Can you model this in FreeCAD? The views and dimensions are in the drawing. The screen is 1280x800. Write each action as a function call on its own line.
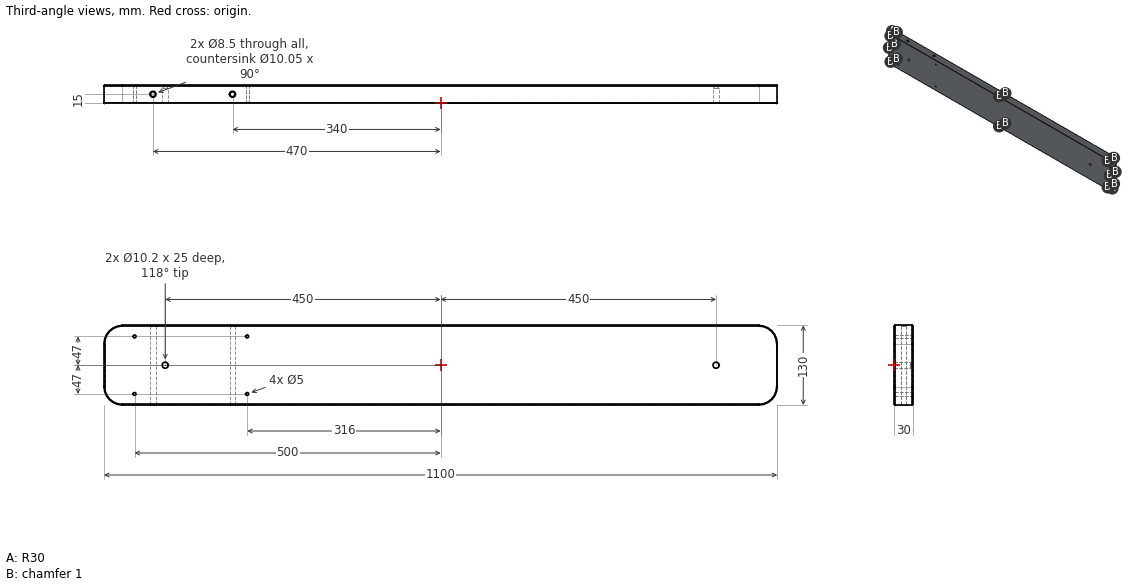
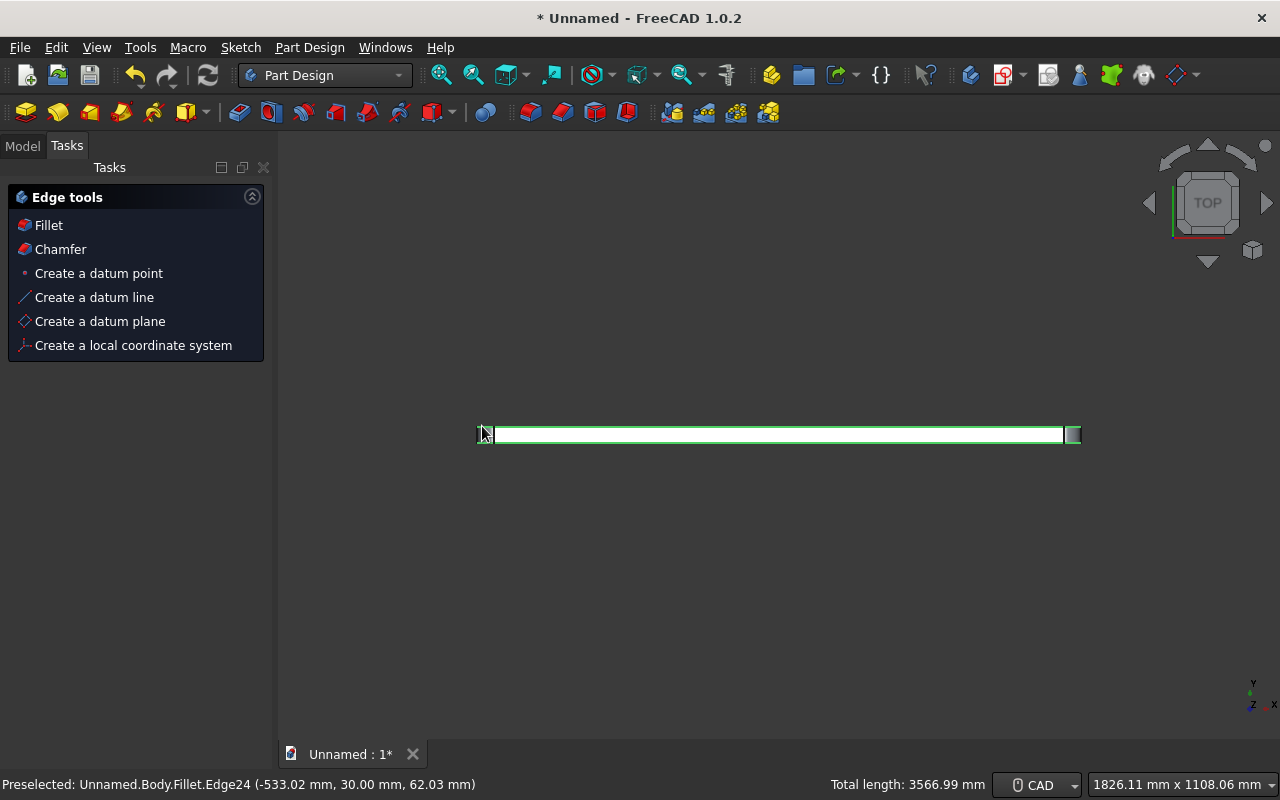
key(1)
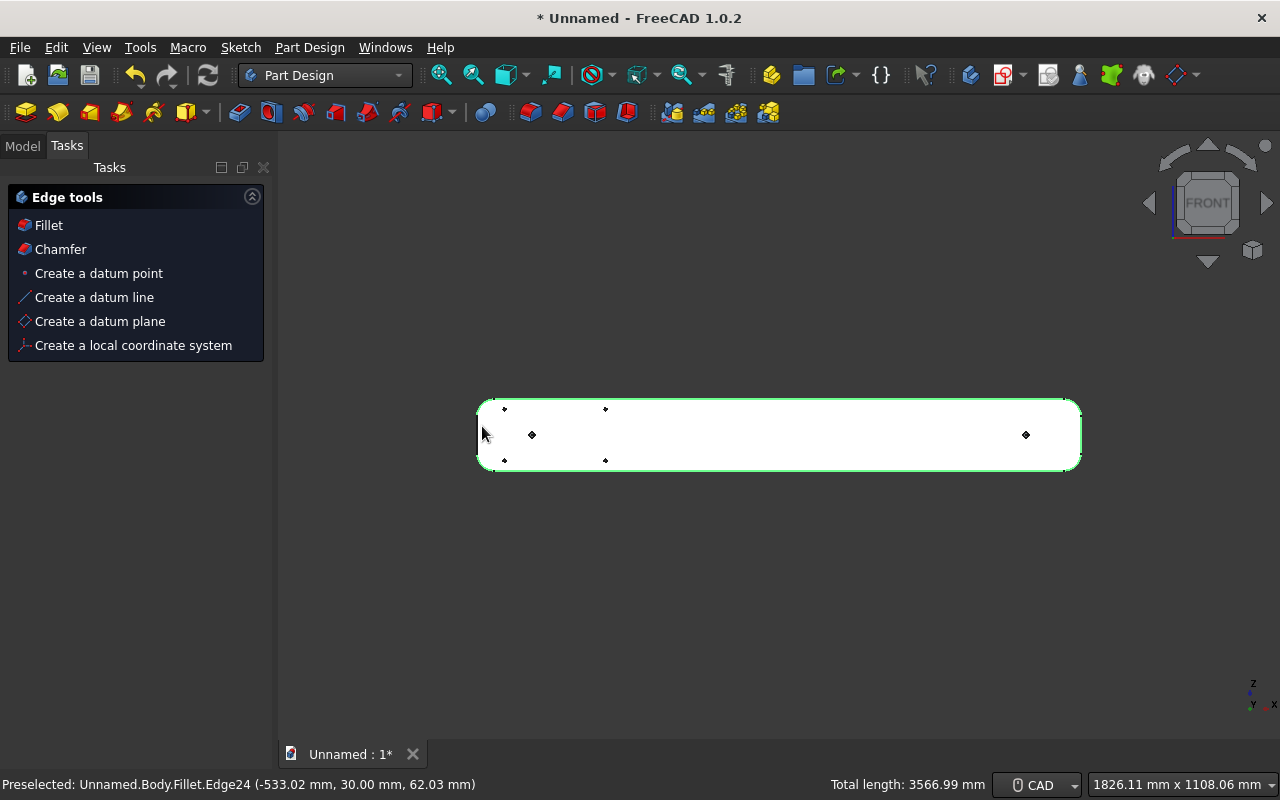
key(3)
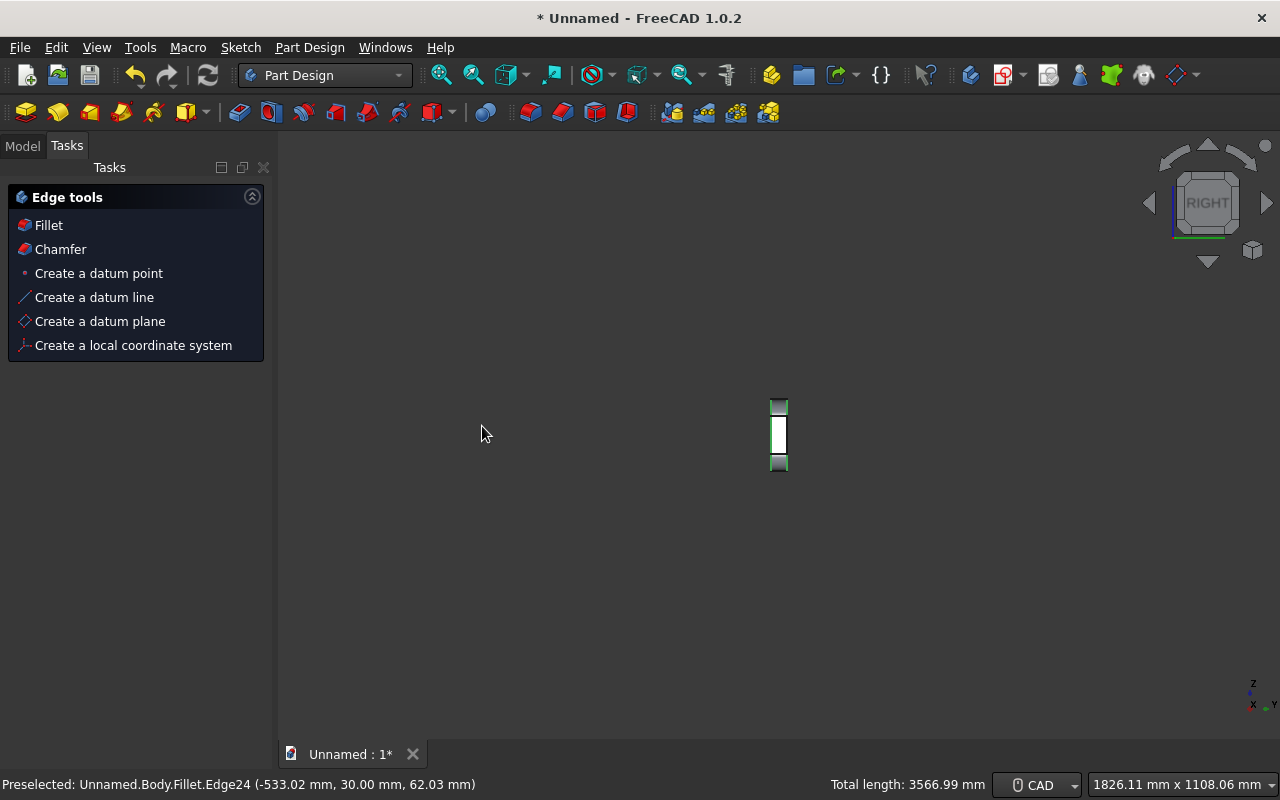
click(442, 76)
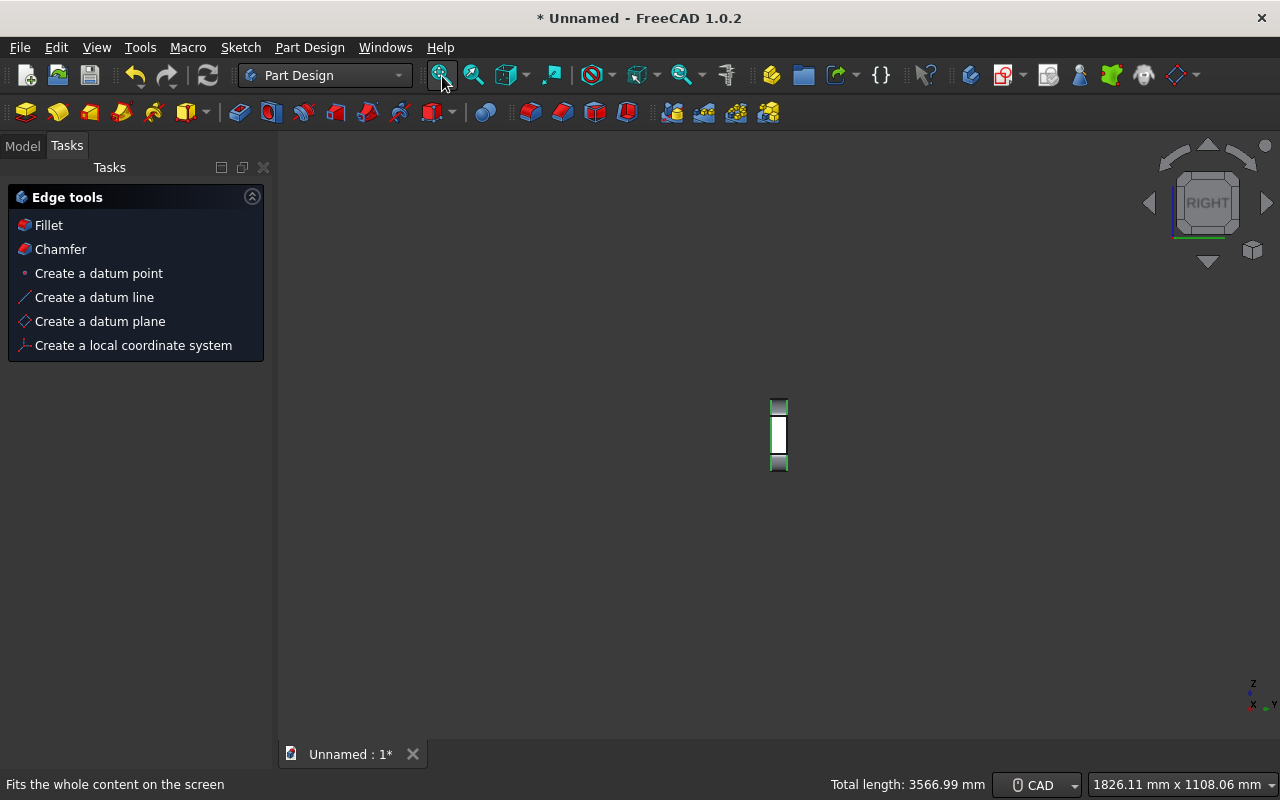
click(787, 434, ctrl)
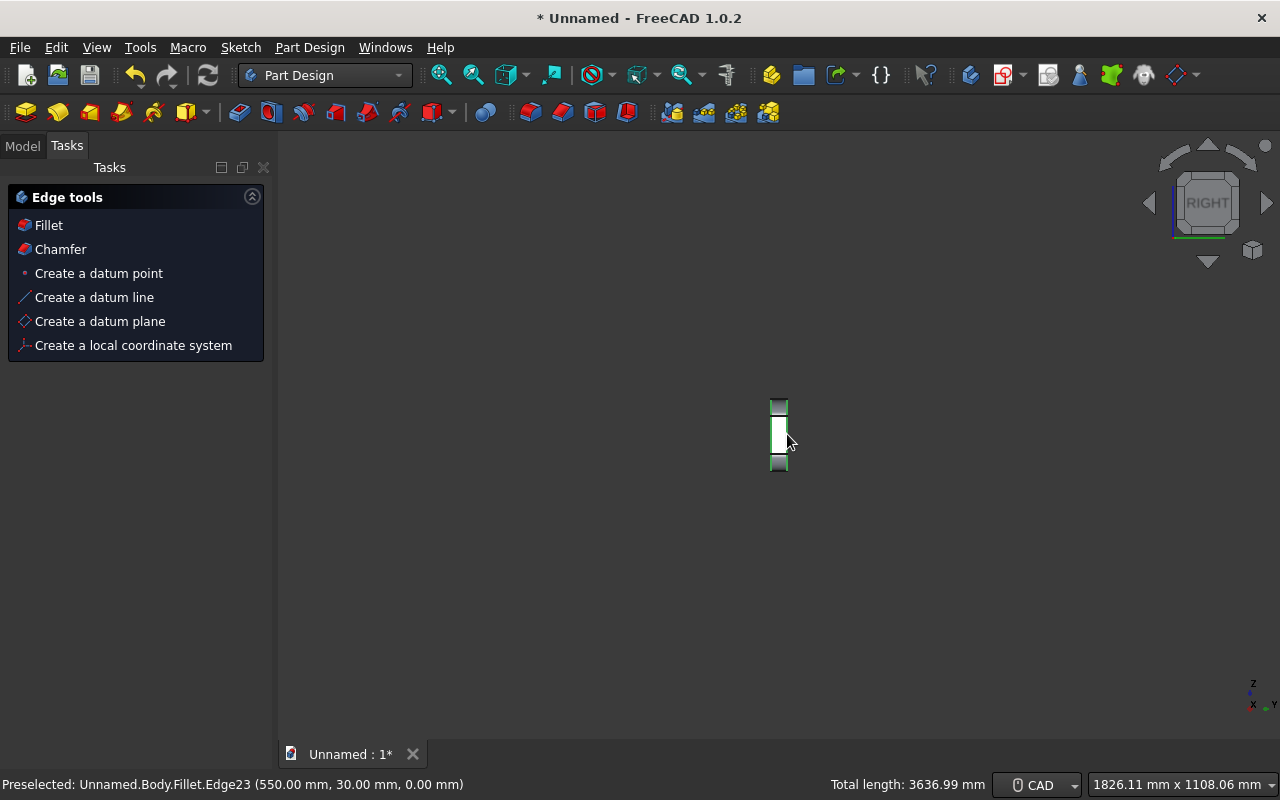
key(5)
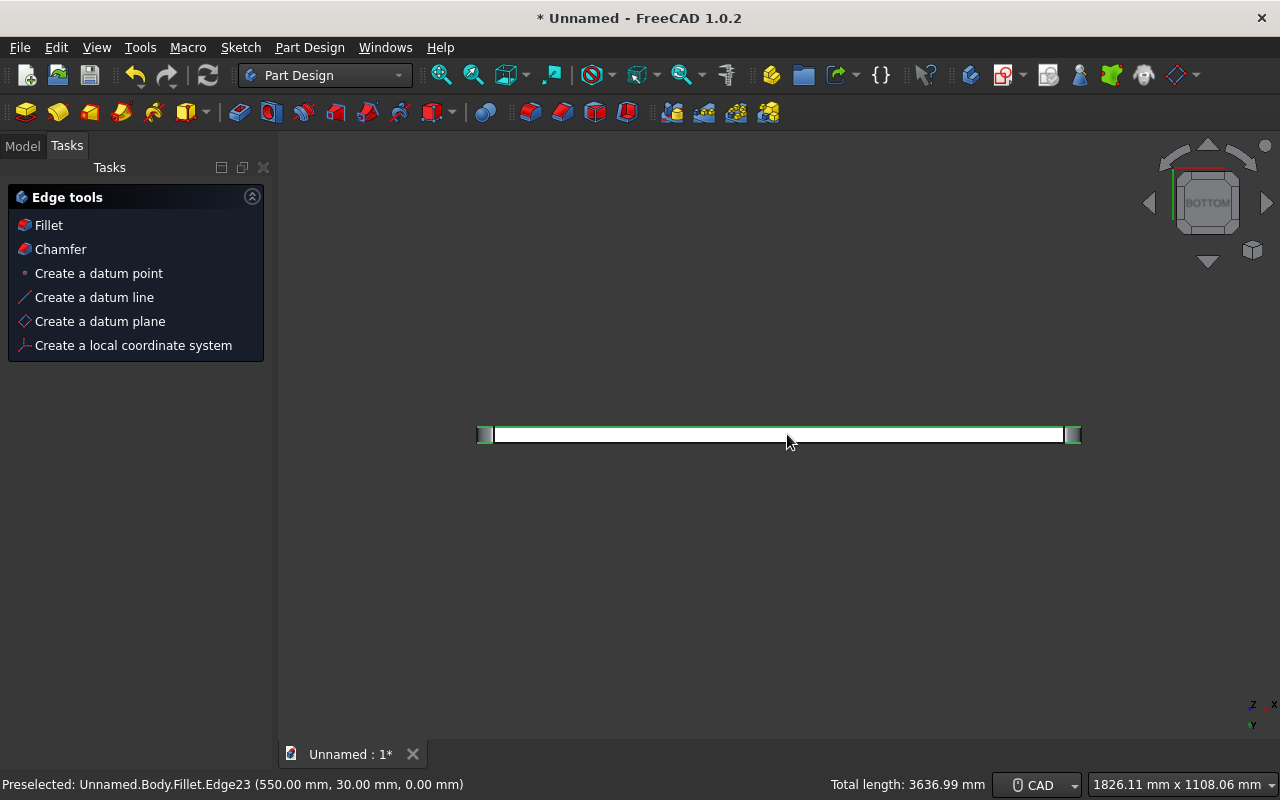
key(4)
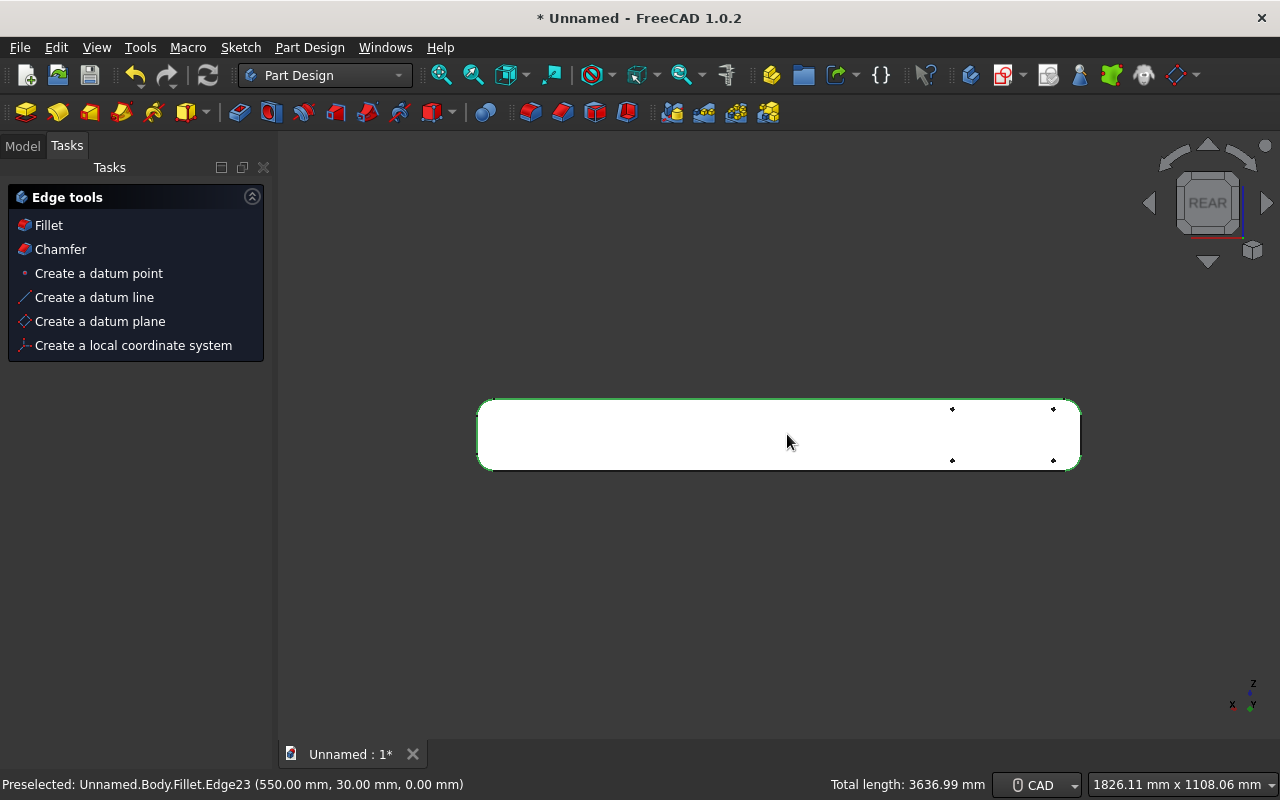
click(1081, 434, ctrl)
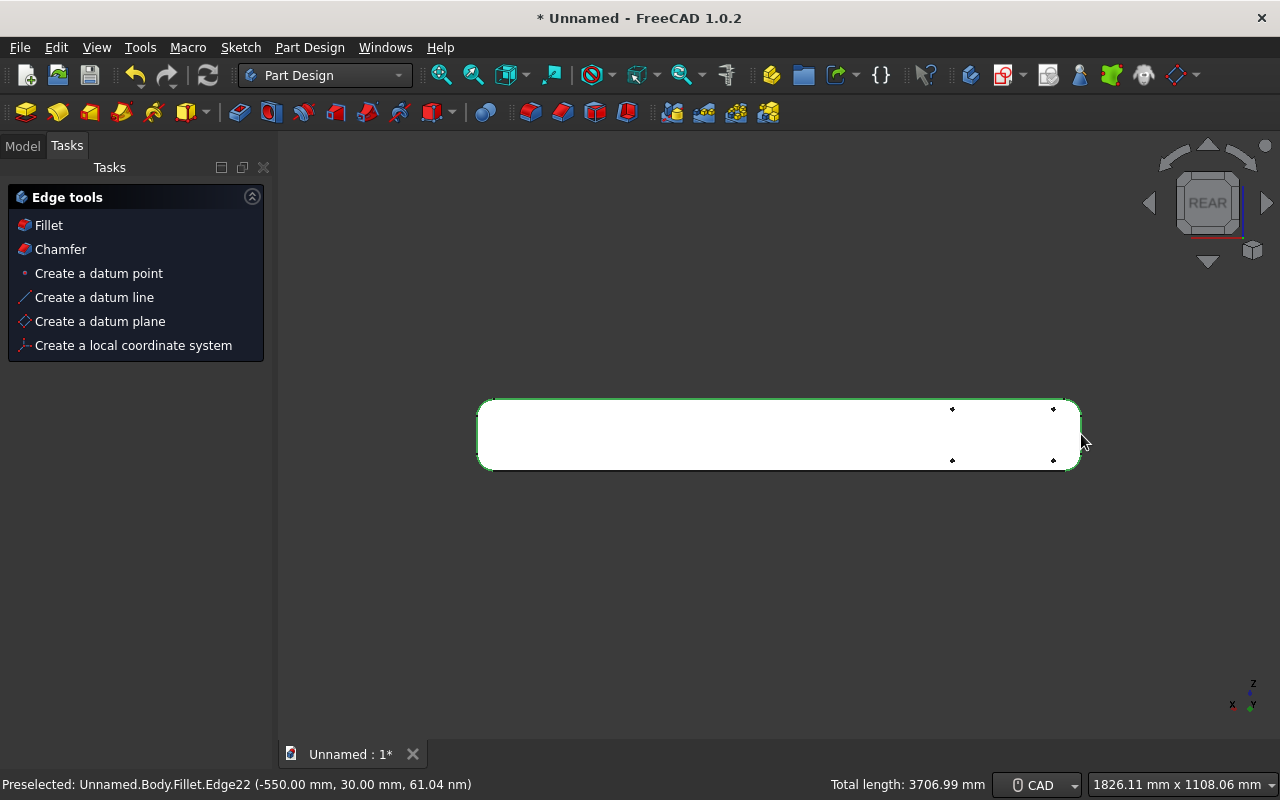
click(779, 470, ctrl)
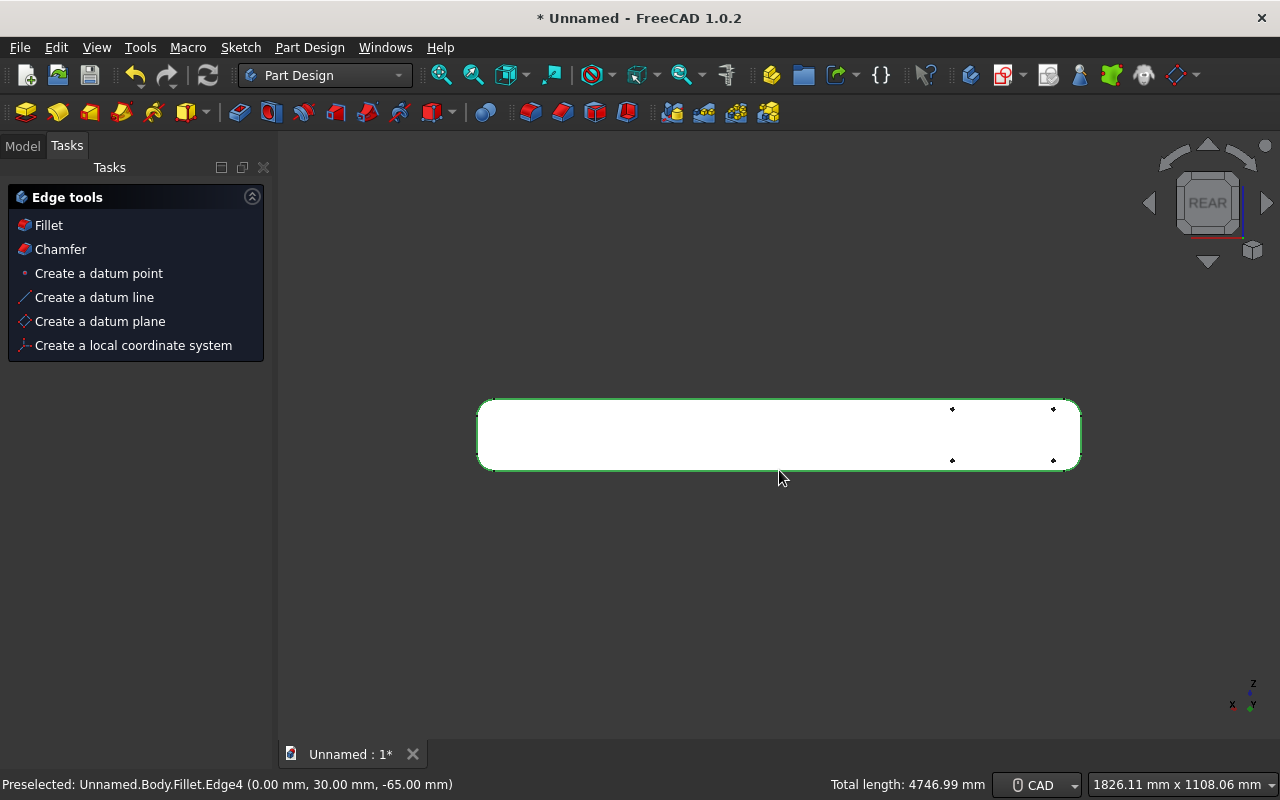
key(6)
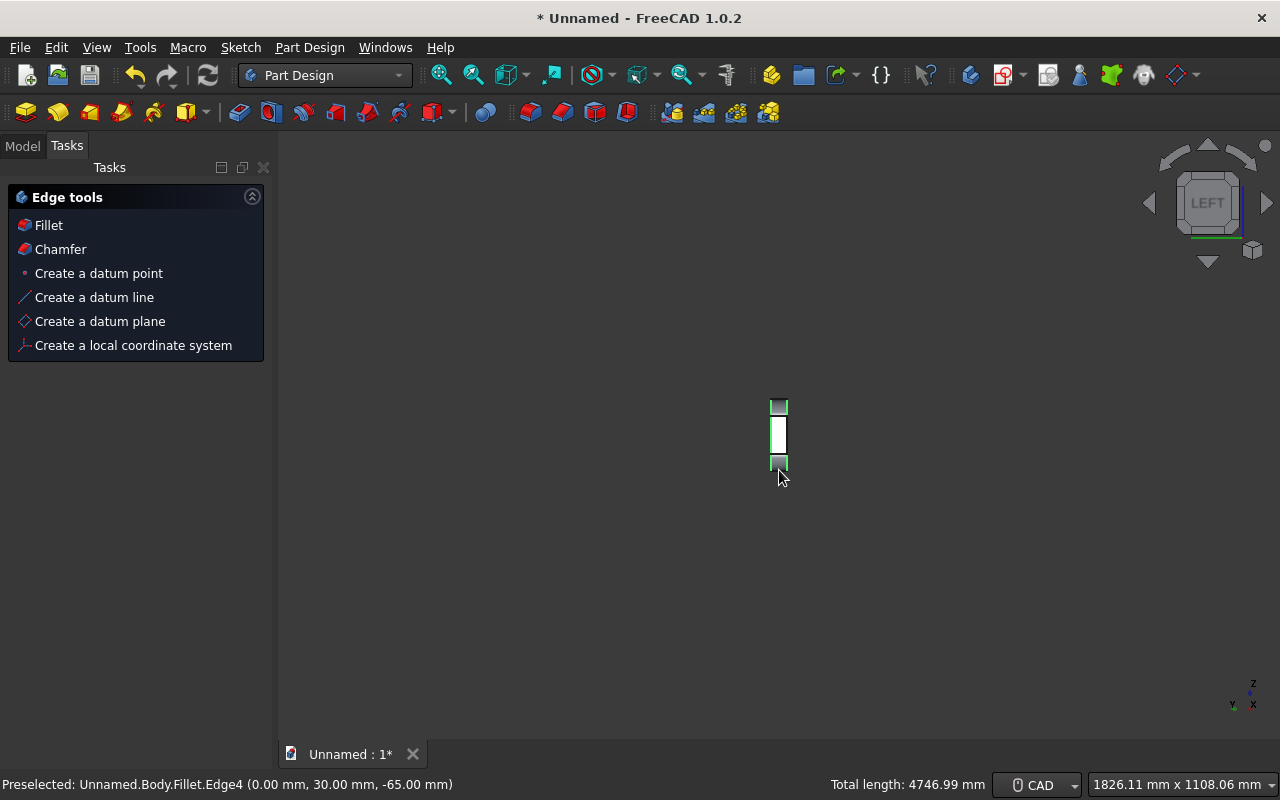
click(442, 76)